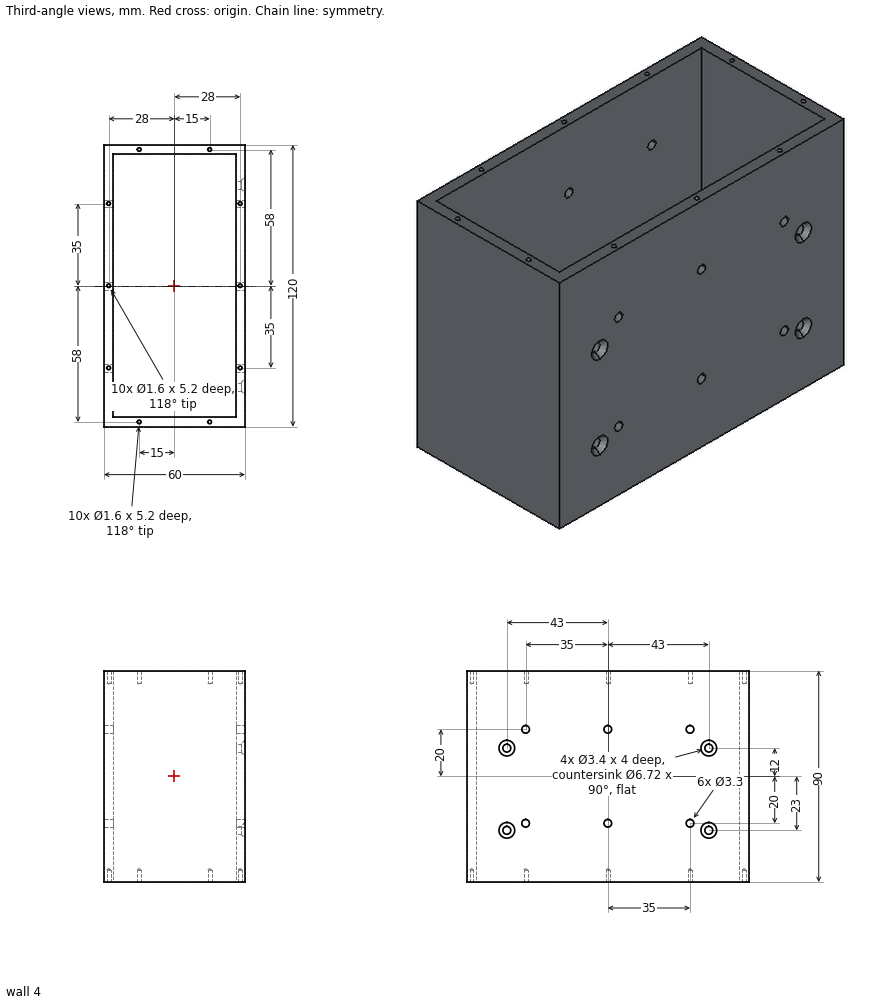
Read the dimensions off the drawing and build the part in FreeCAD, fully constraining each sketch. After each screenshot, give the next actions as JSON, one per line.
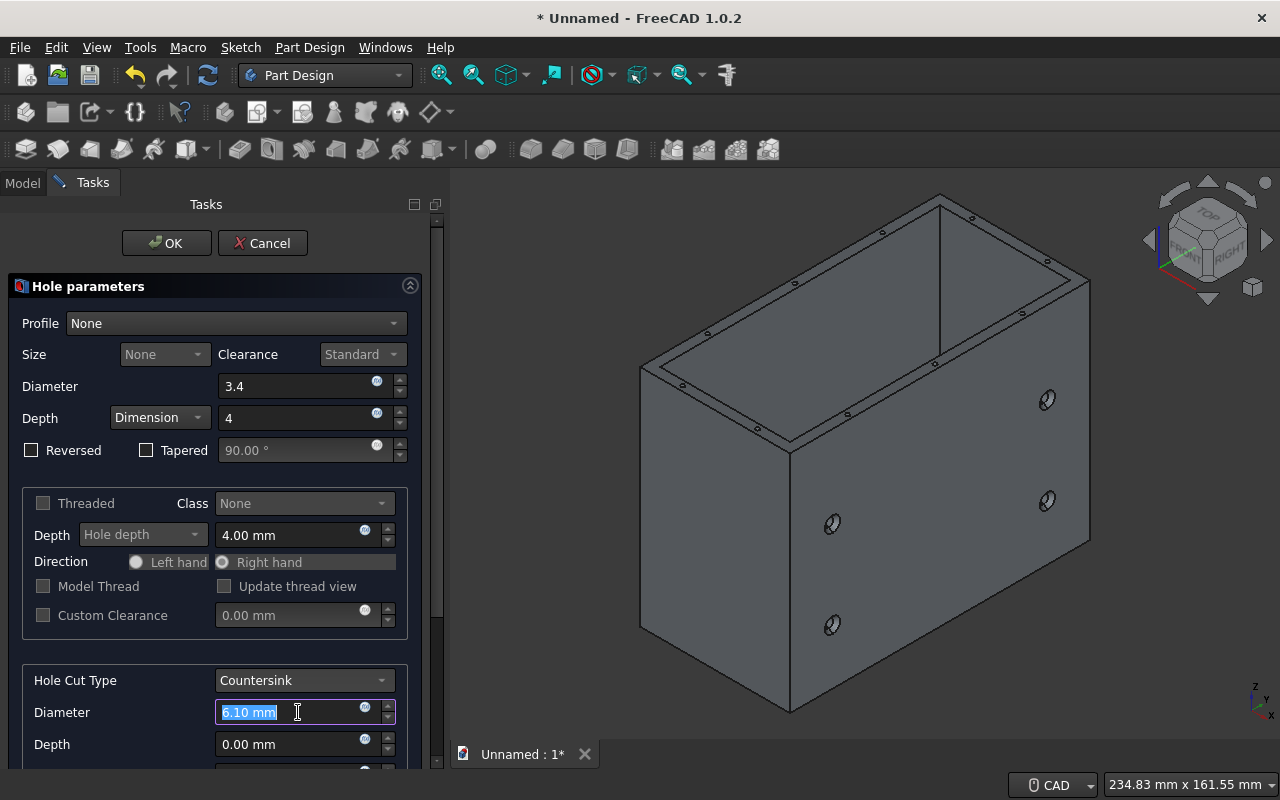
{"action": "type", "text": "6.72"}
{"action": "key", "text": "Tab"}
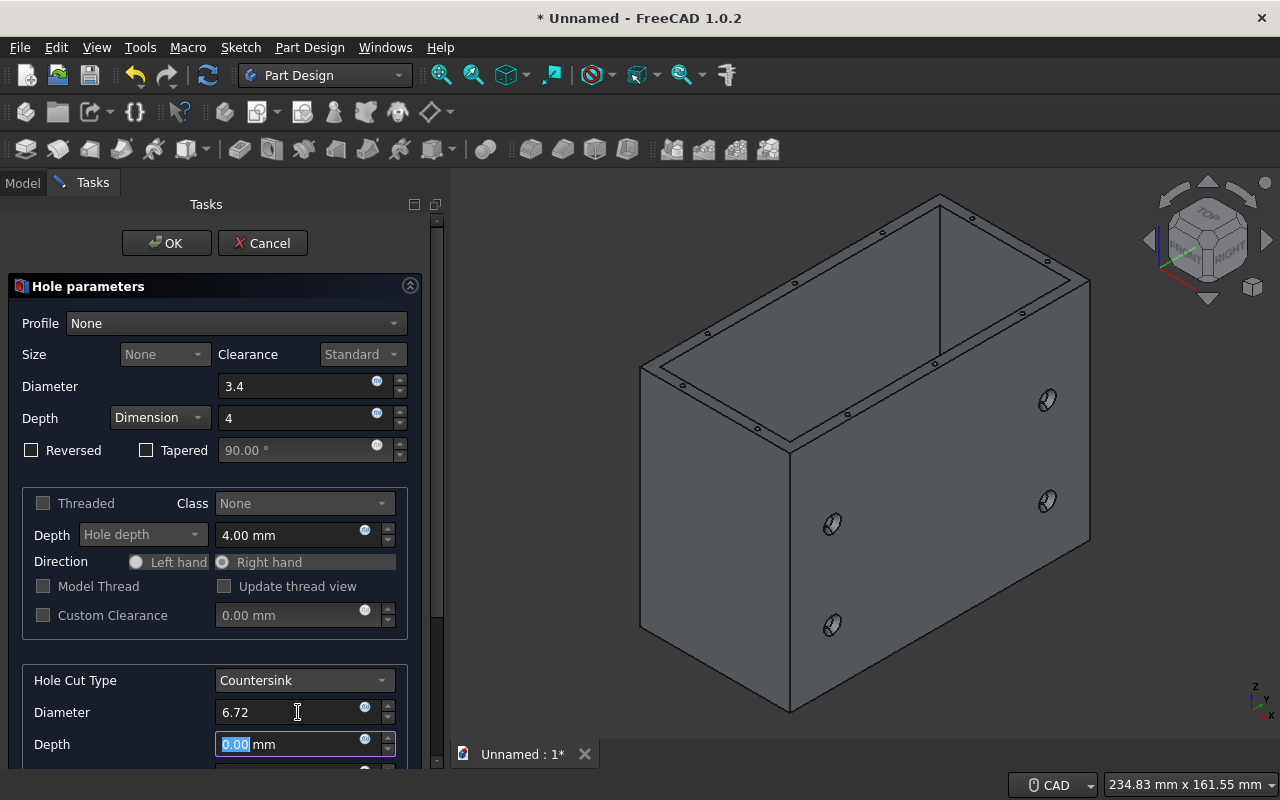
{"action": "scroll", "coordinate": [437, 491], "scroll_direction": "down", "scroll_amount": 3}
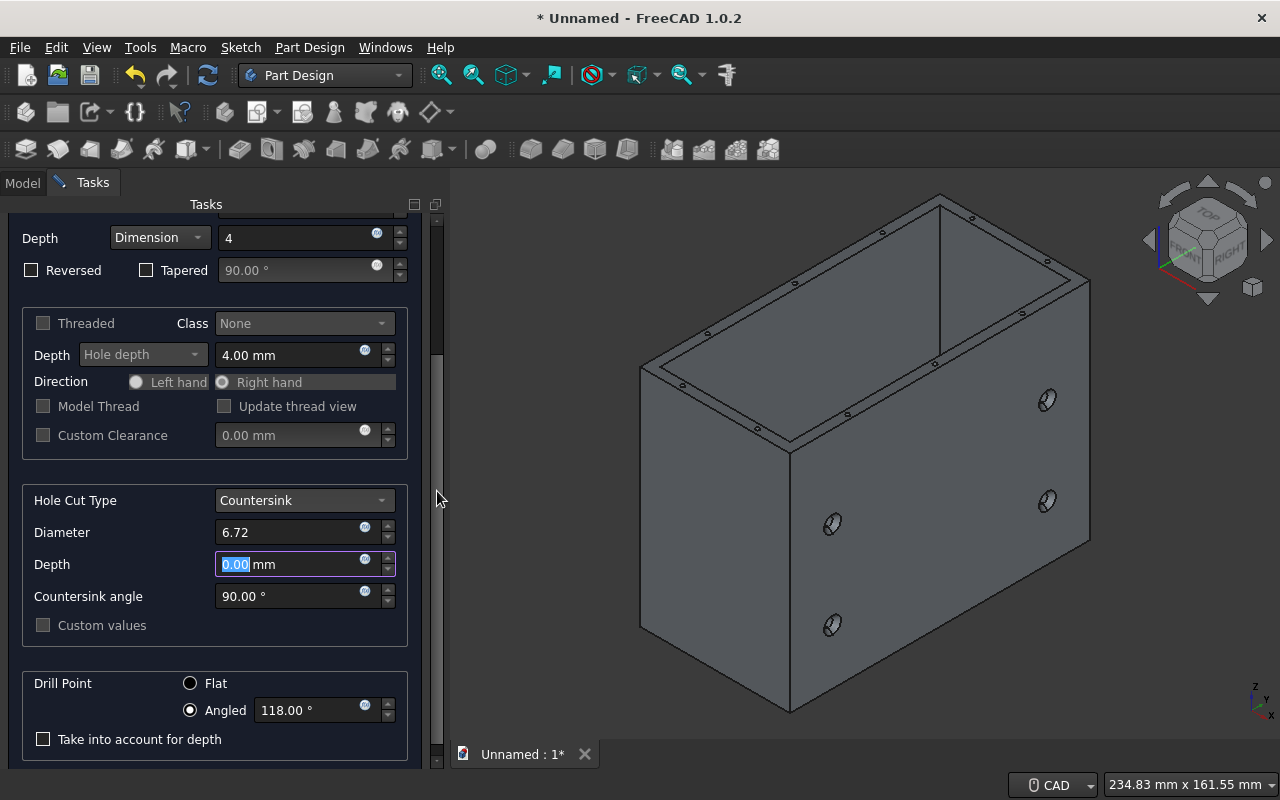
{"action": "left_click", "coordinate": [191, 683]}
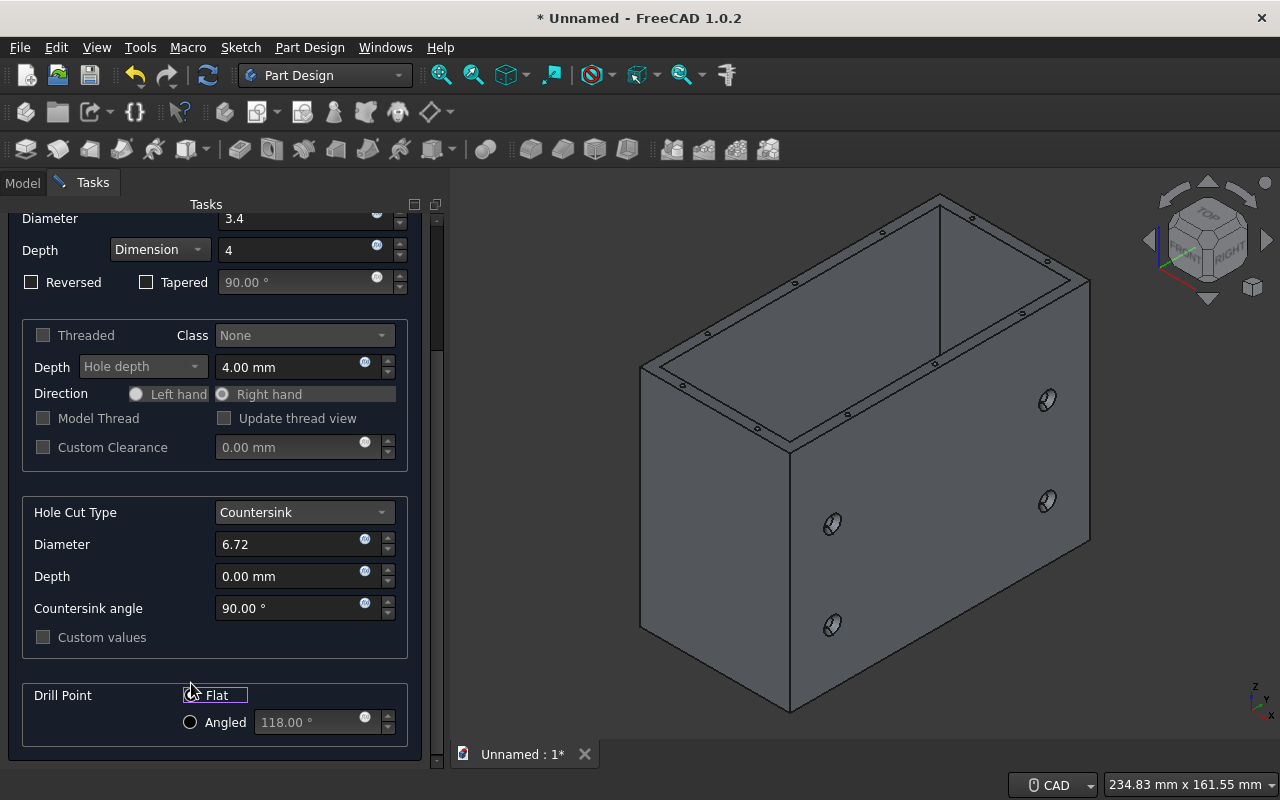
{"action": "scroll", "coordinate": [437, 491], "scroll_direction": "up", "scroll_amount": 4}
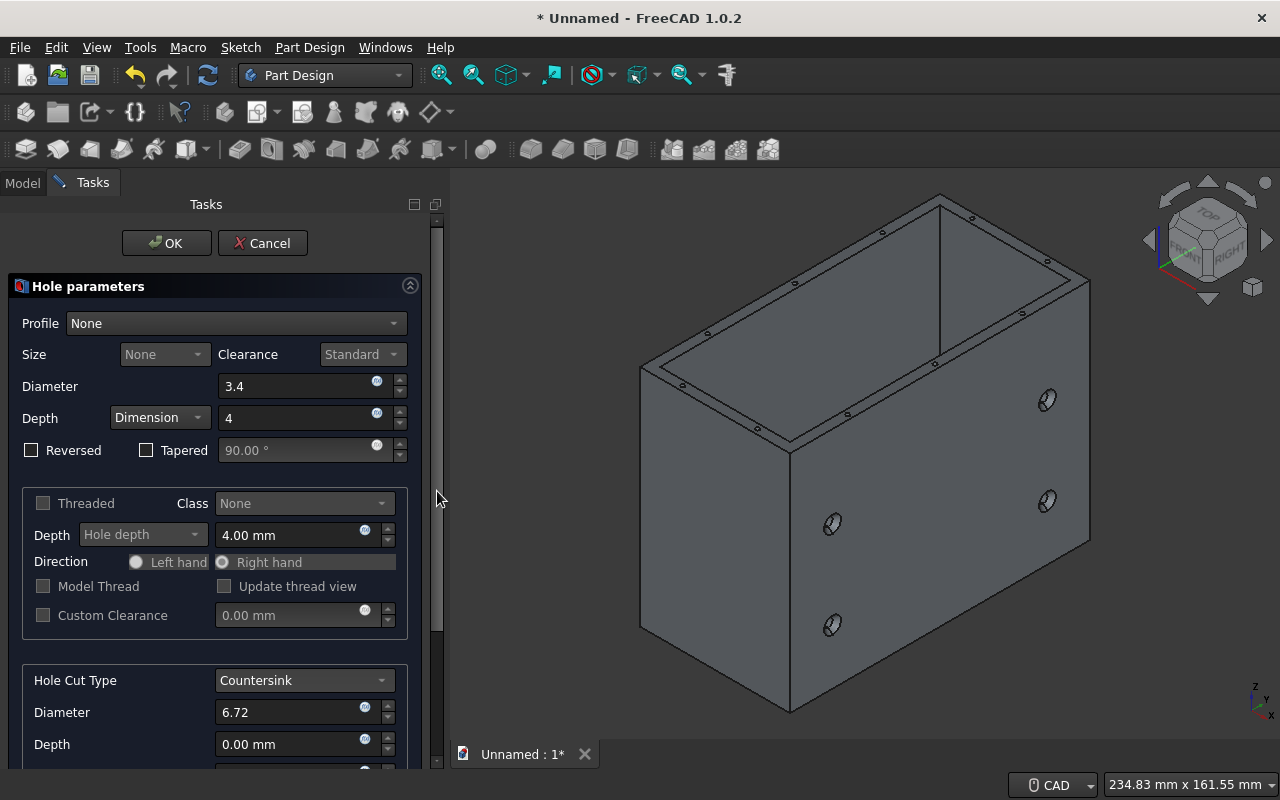
{"action": "left_click", "coordinate": [167, 243]}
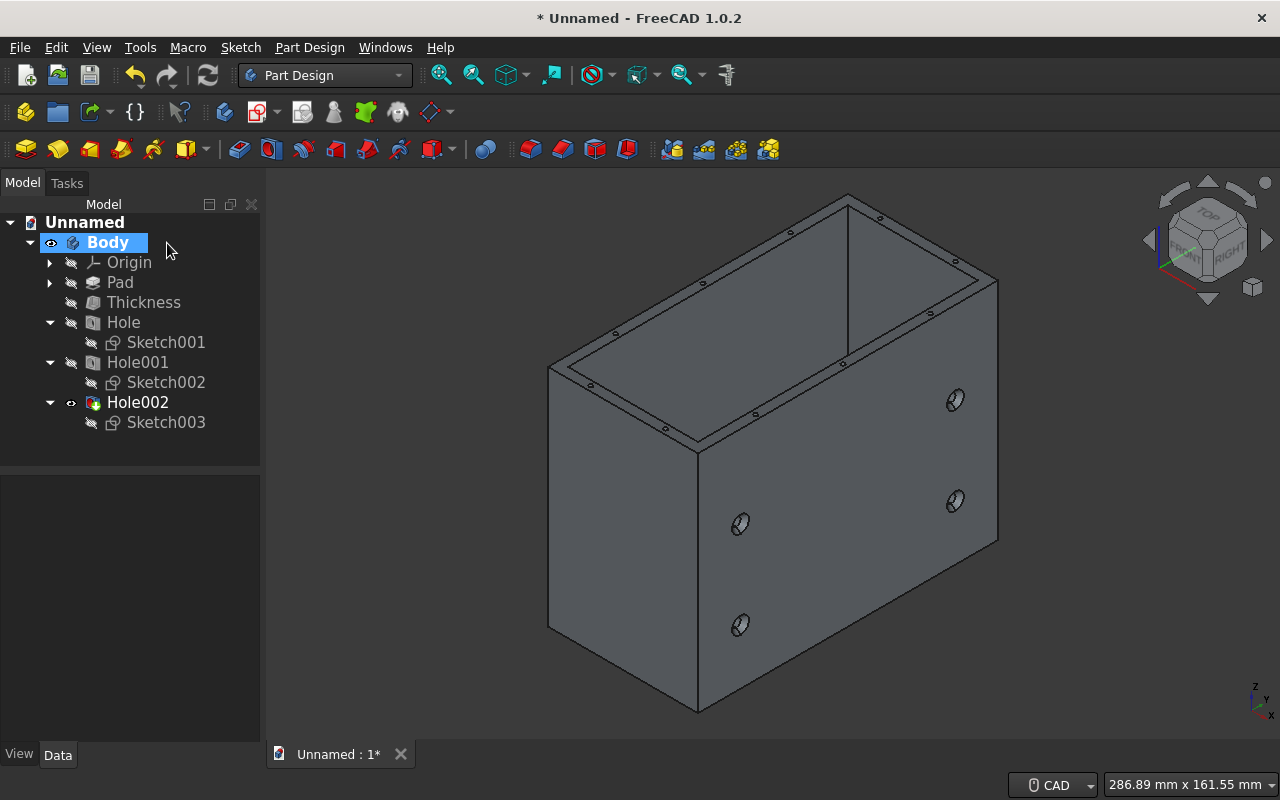
{"action": "left_click", "coordinate": [848, 496]}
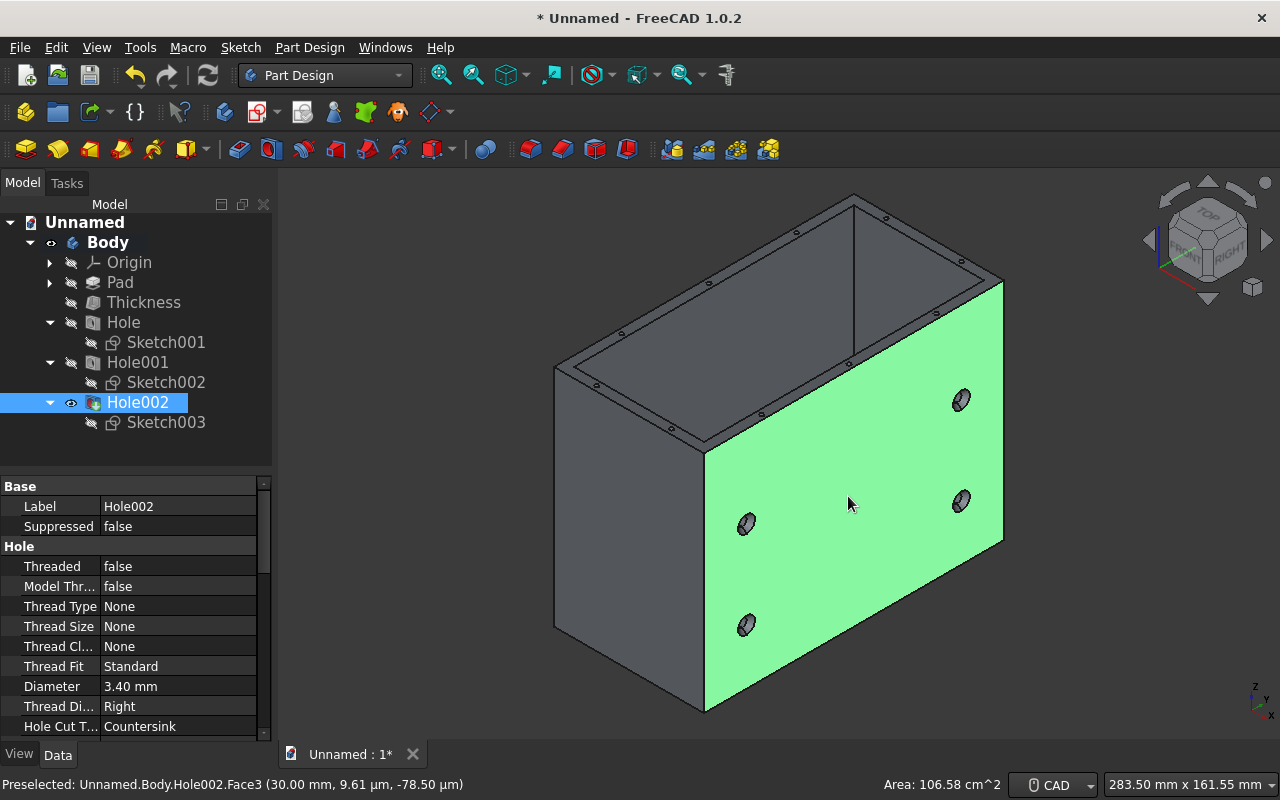
{"action": "left_click", "coordinate": [258, 112]}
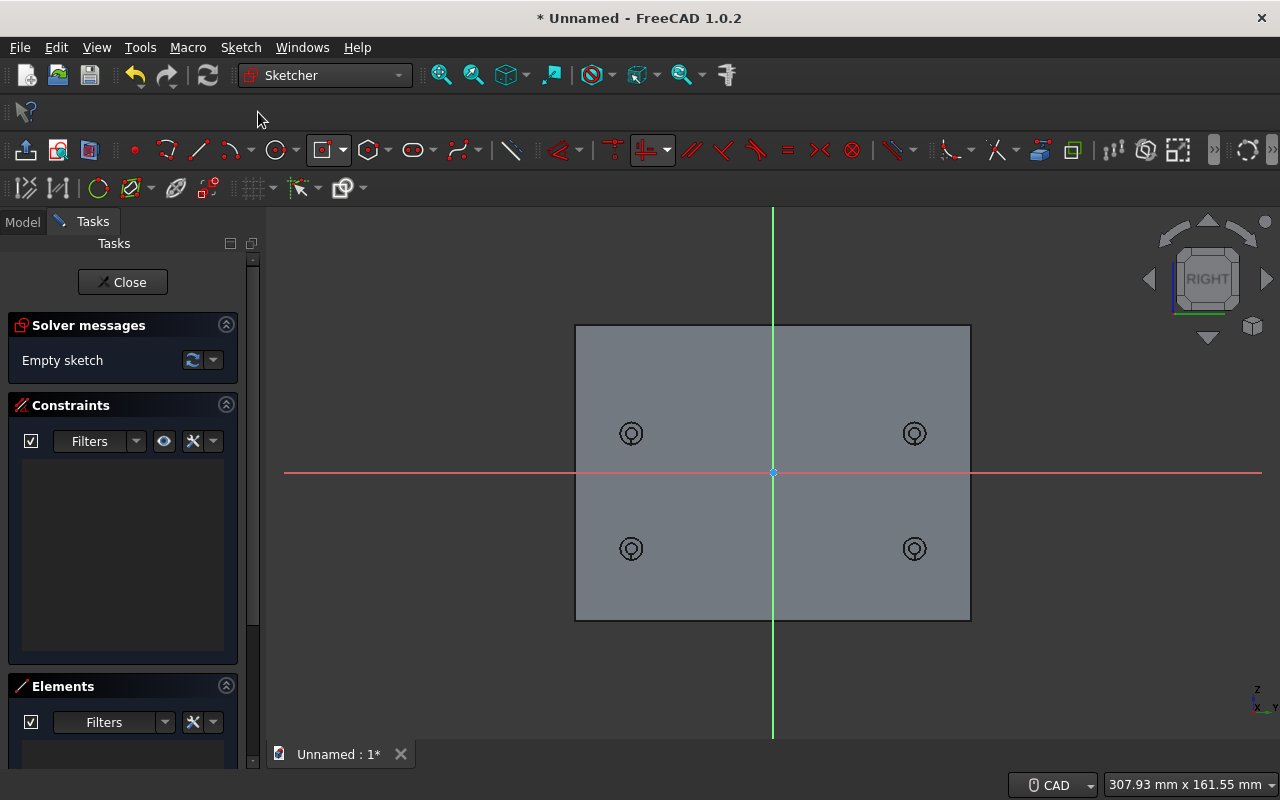
{"action": "scroll", "coordinate": [829, 473], "scroll_direction": "up", "scroll_amount": 4}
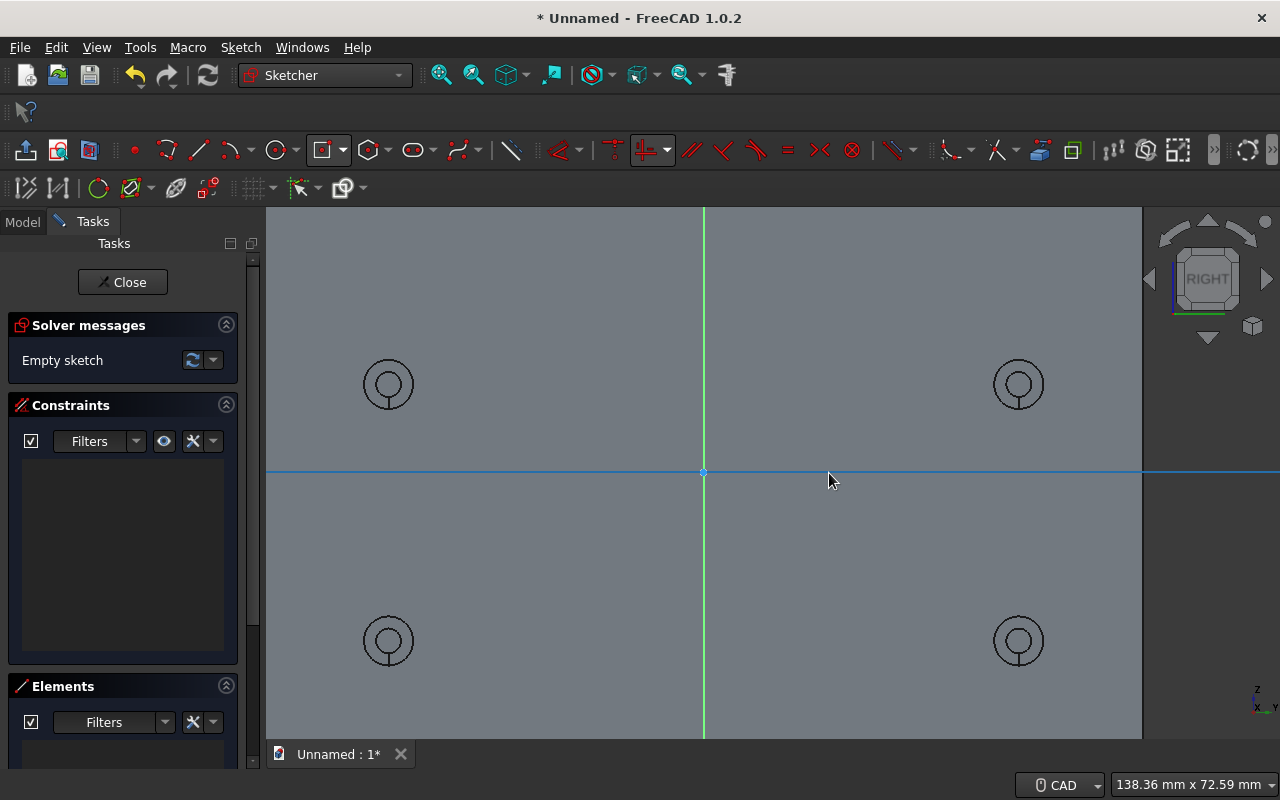
{"action": "left_click", "coordinate": [276, 150]}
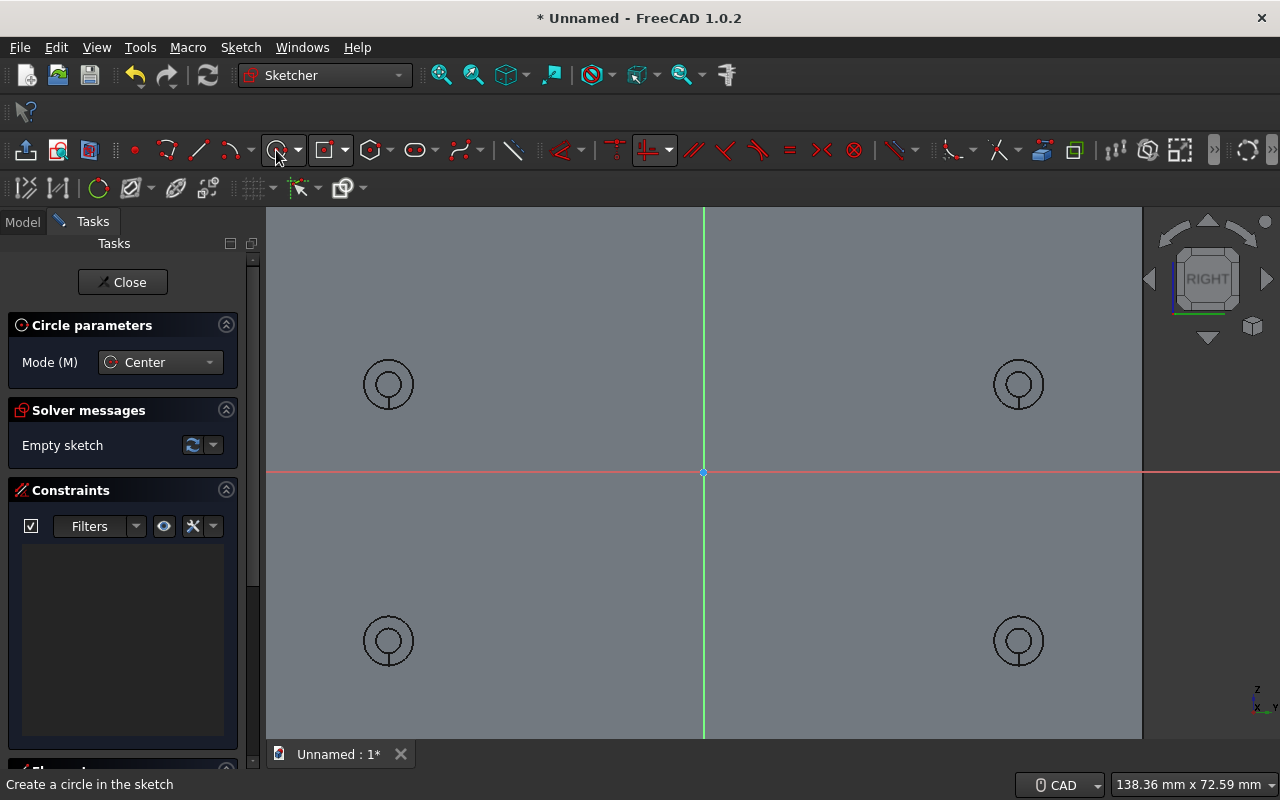
{"action": "scroll", "coordinate": [960, 619], "scroll_direction": "up", "scroll_amount": 4}